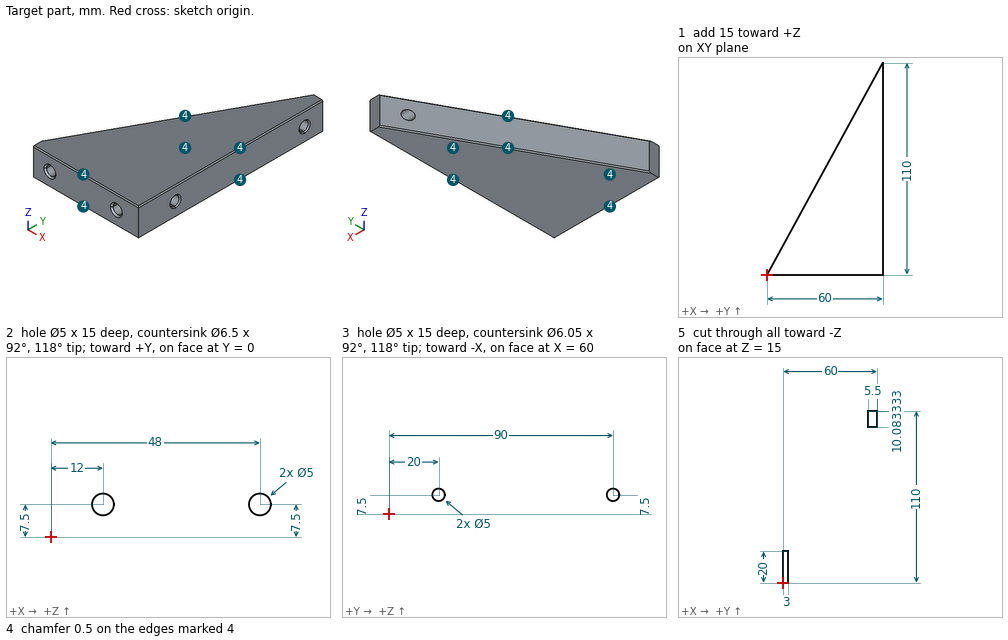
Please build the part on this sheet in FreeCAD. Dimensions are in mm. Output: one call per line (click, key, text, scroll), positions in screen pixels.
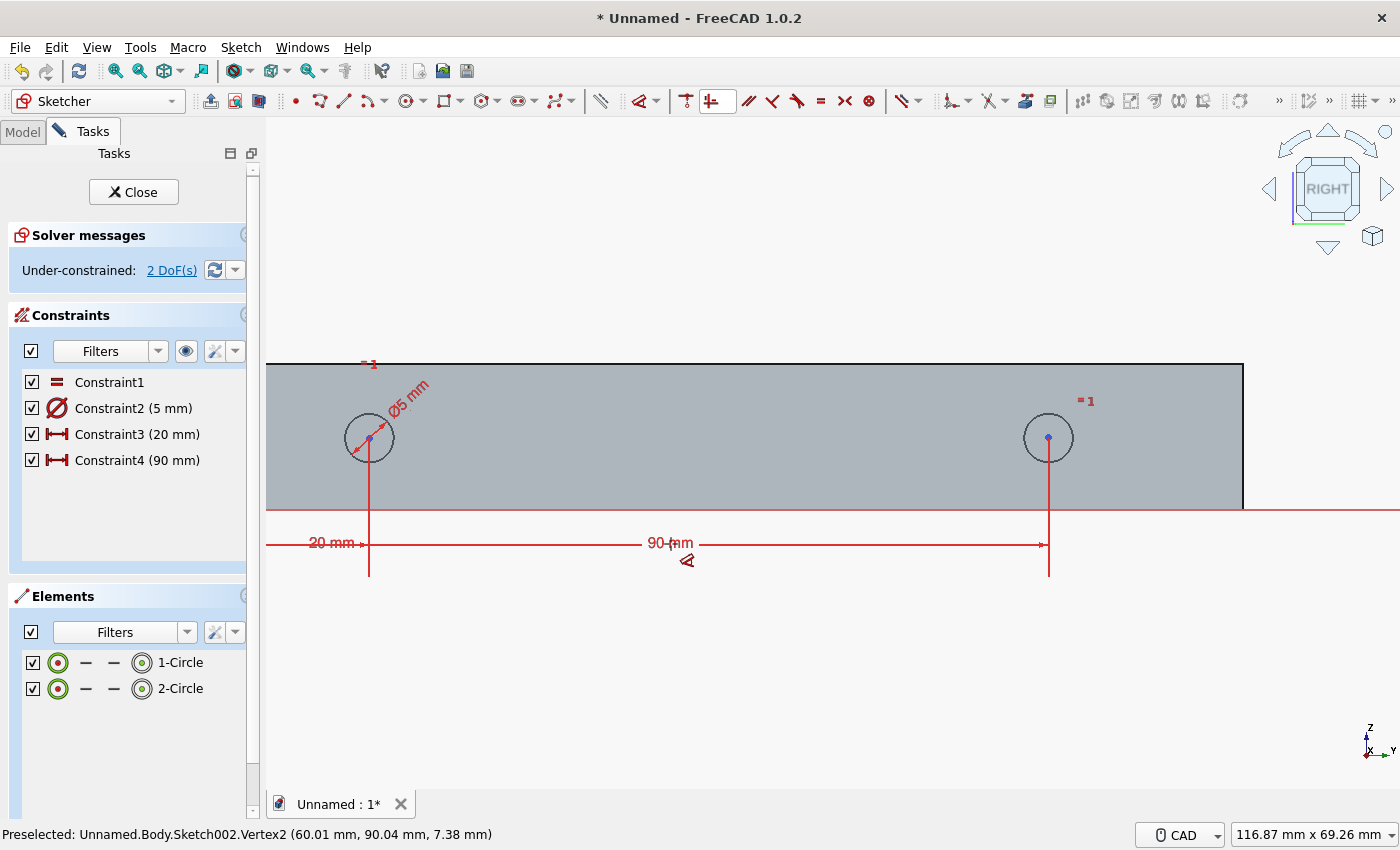
click(369, 438)
click(403, 474)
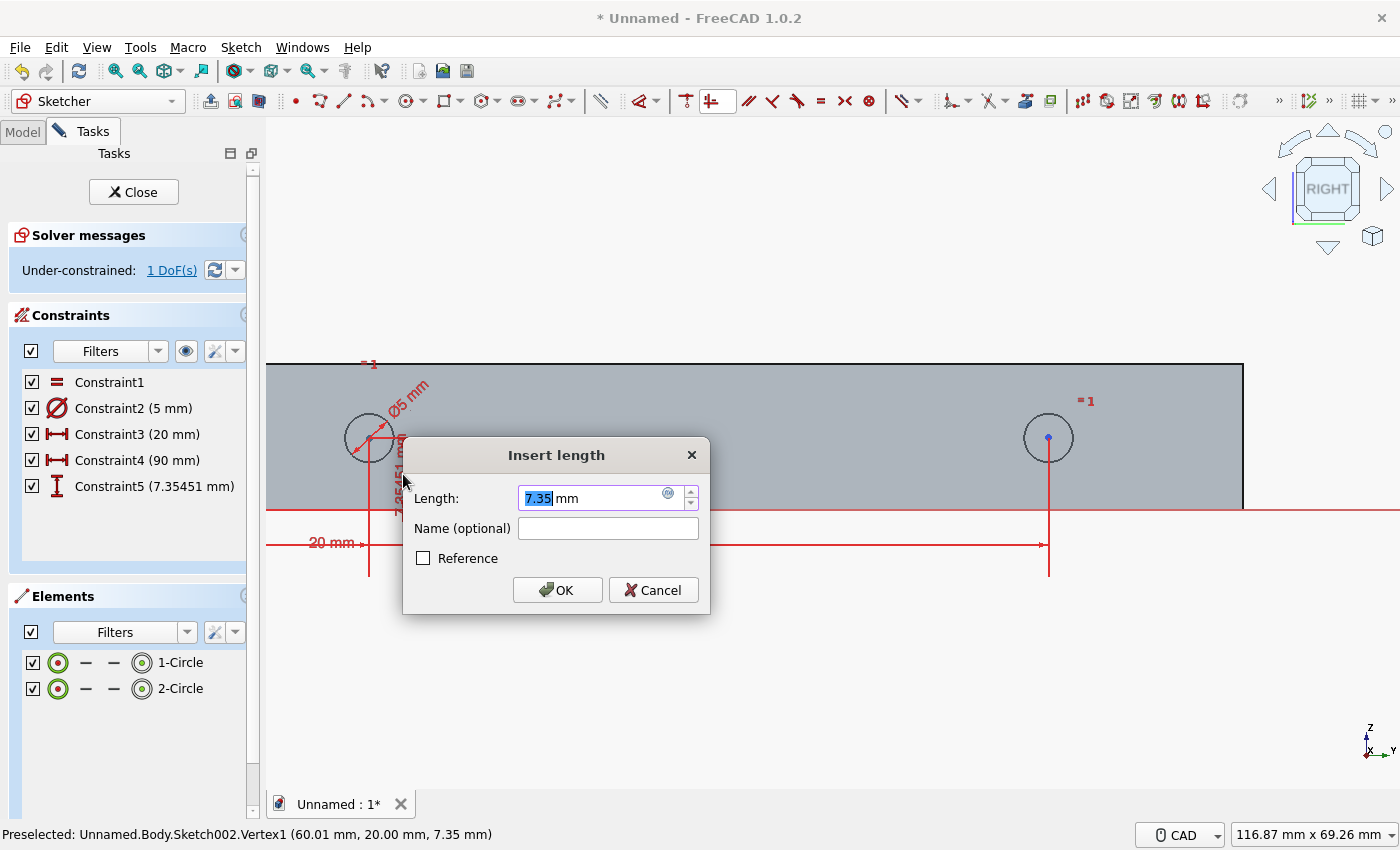
text(7.5)
key(Return)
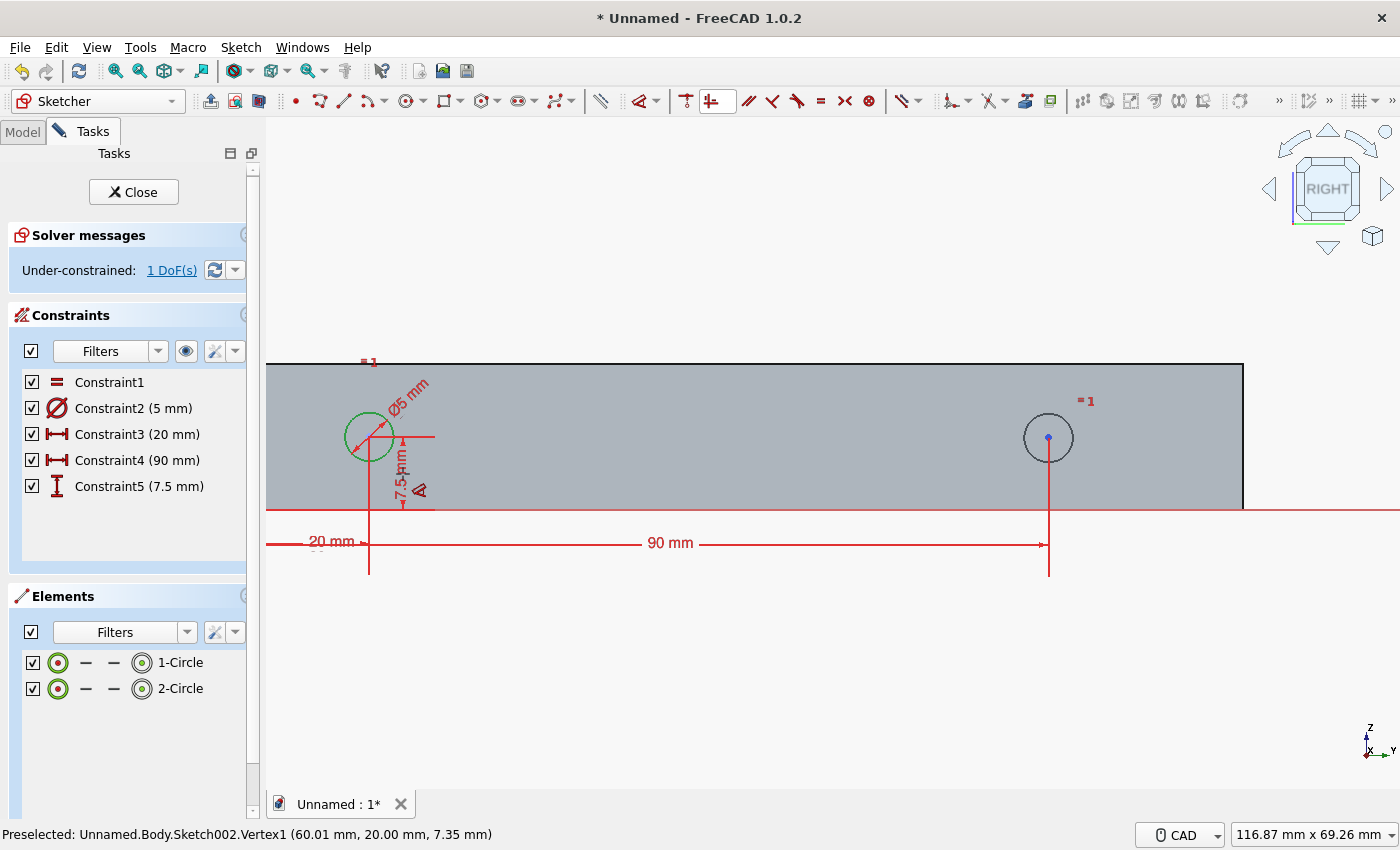
click(1049, 438)
click(1083, 474)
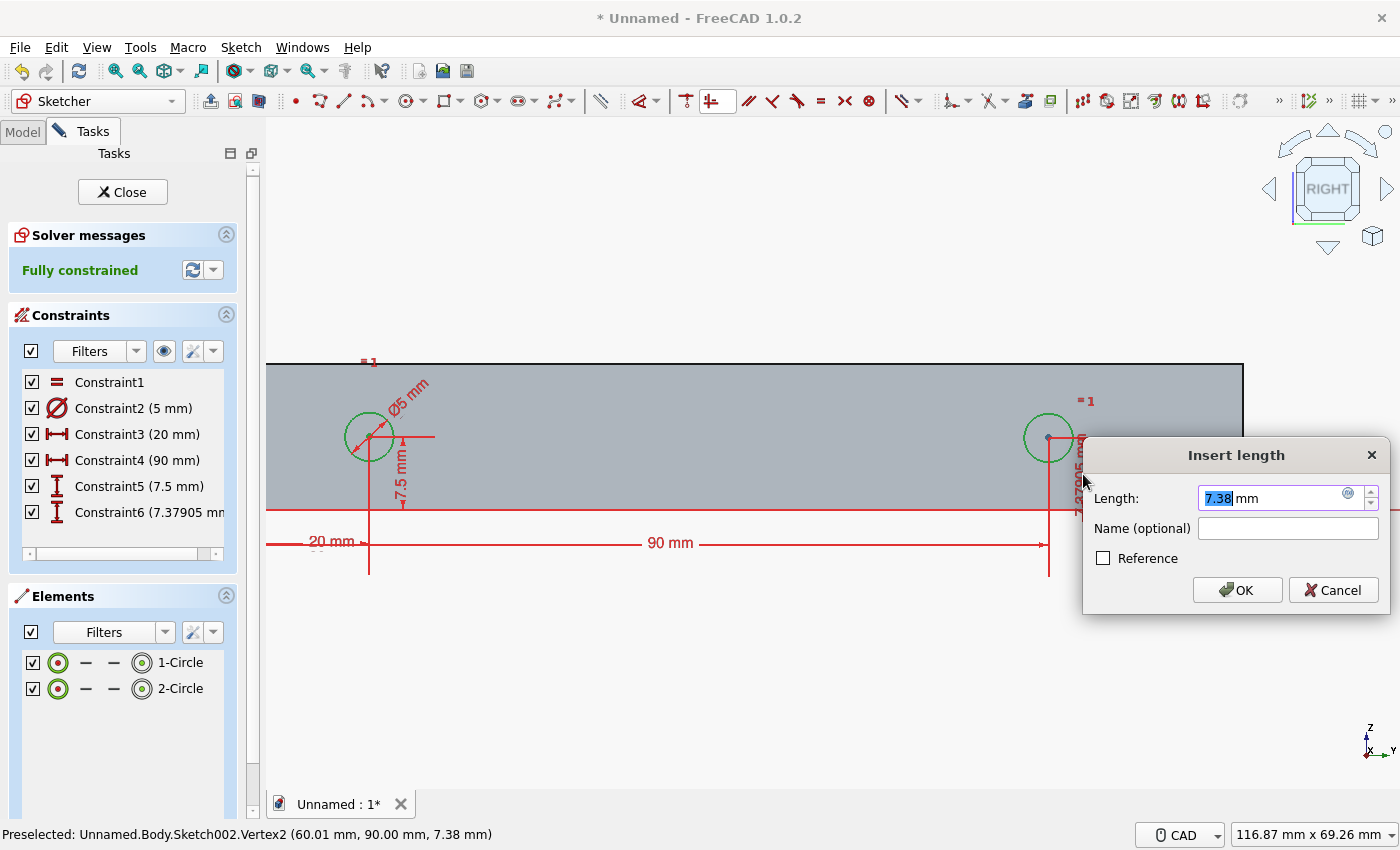
text(7.5)
key(Return)
key(Escape)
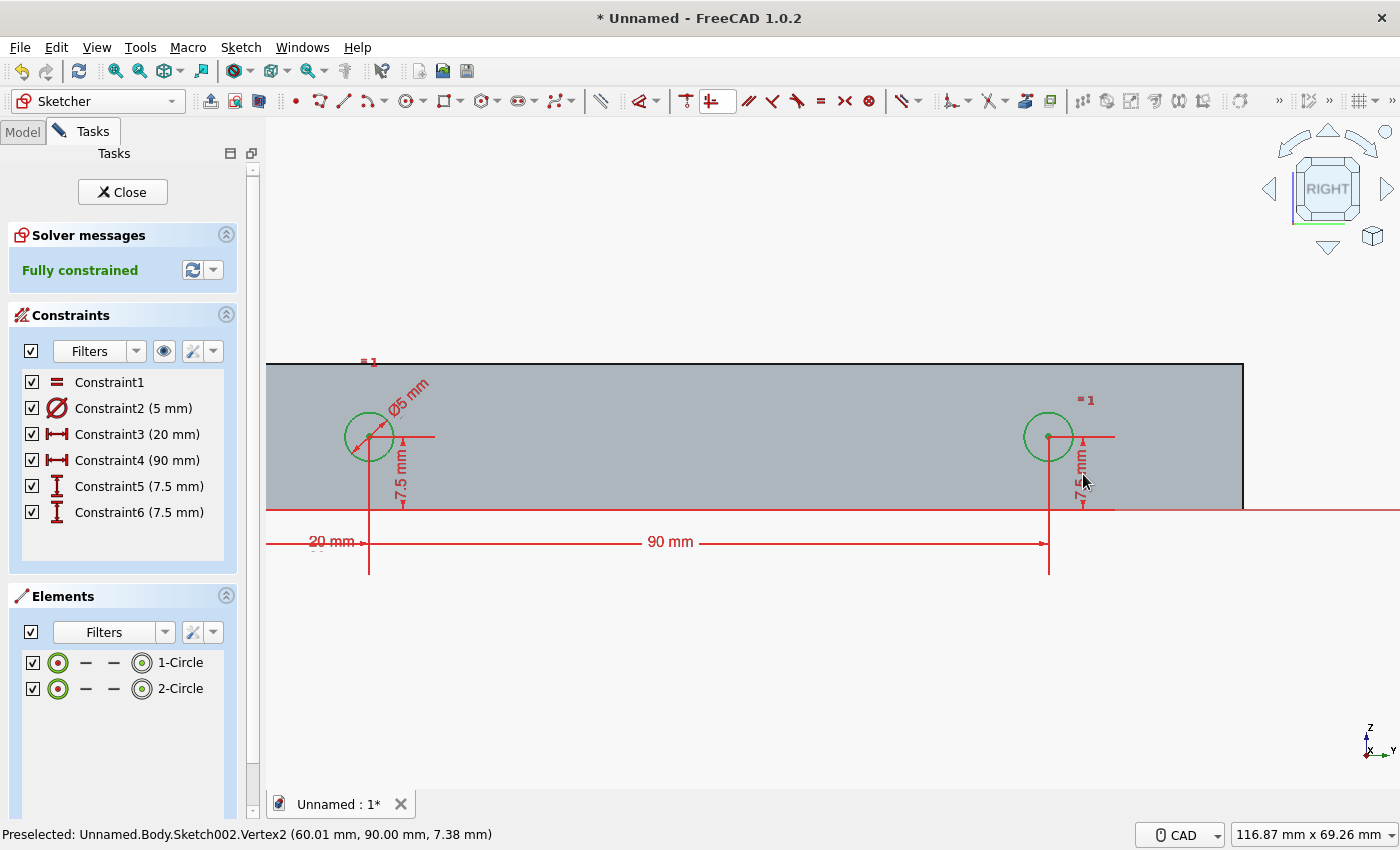
click(123, 192)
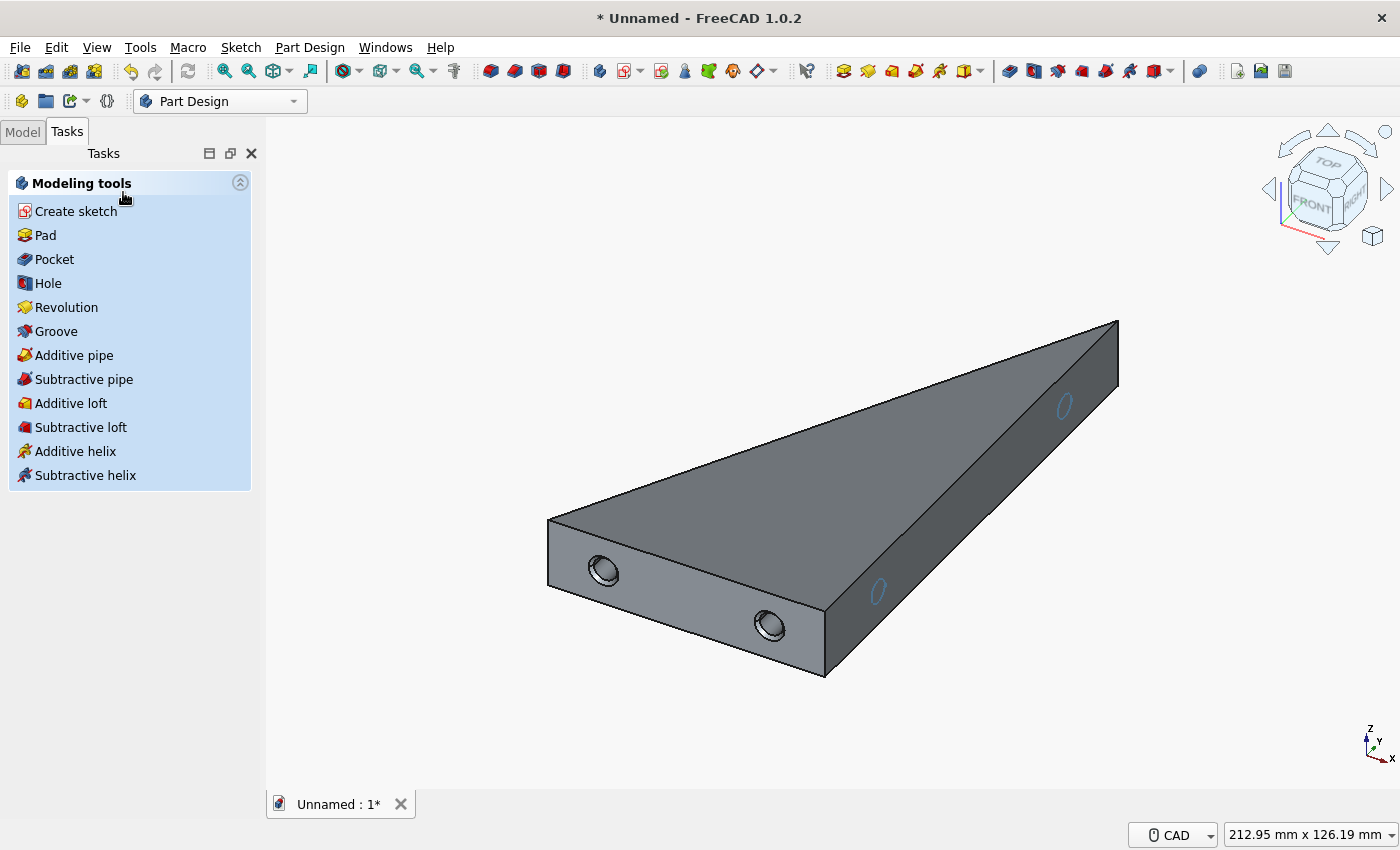
click(1034, 72)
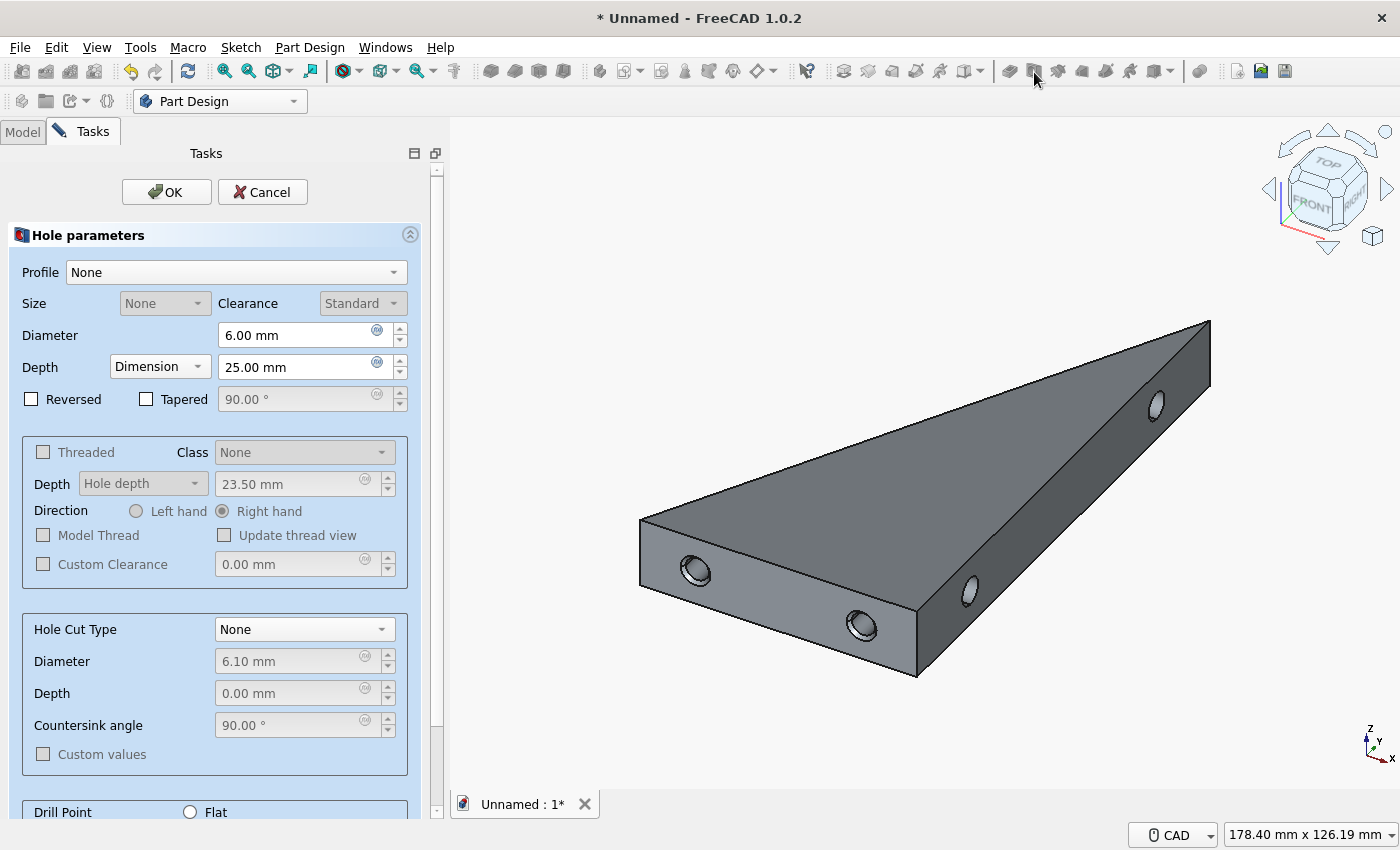
triple_click(305, 335)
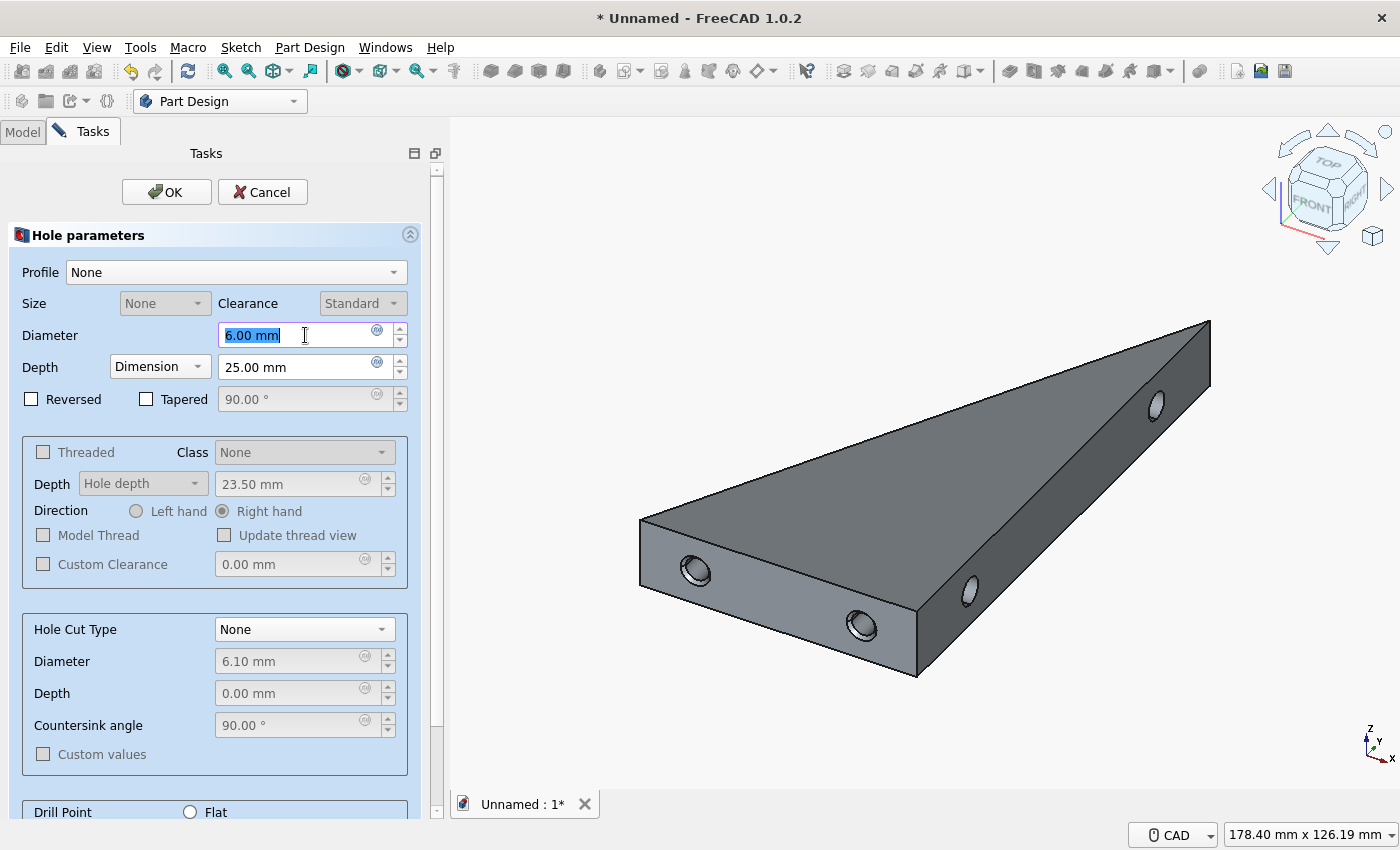
text(5)
key(Tab)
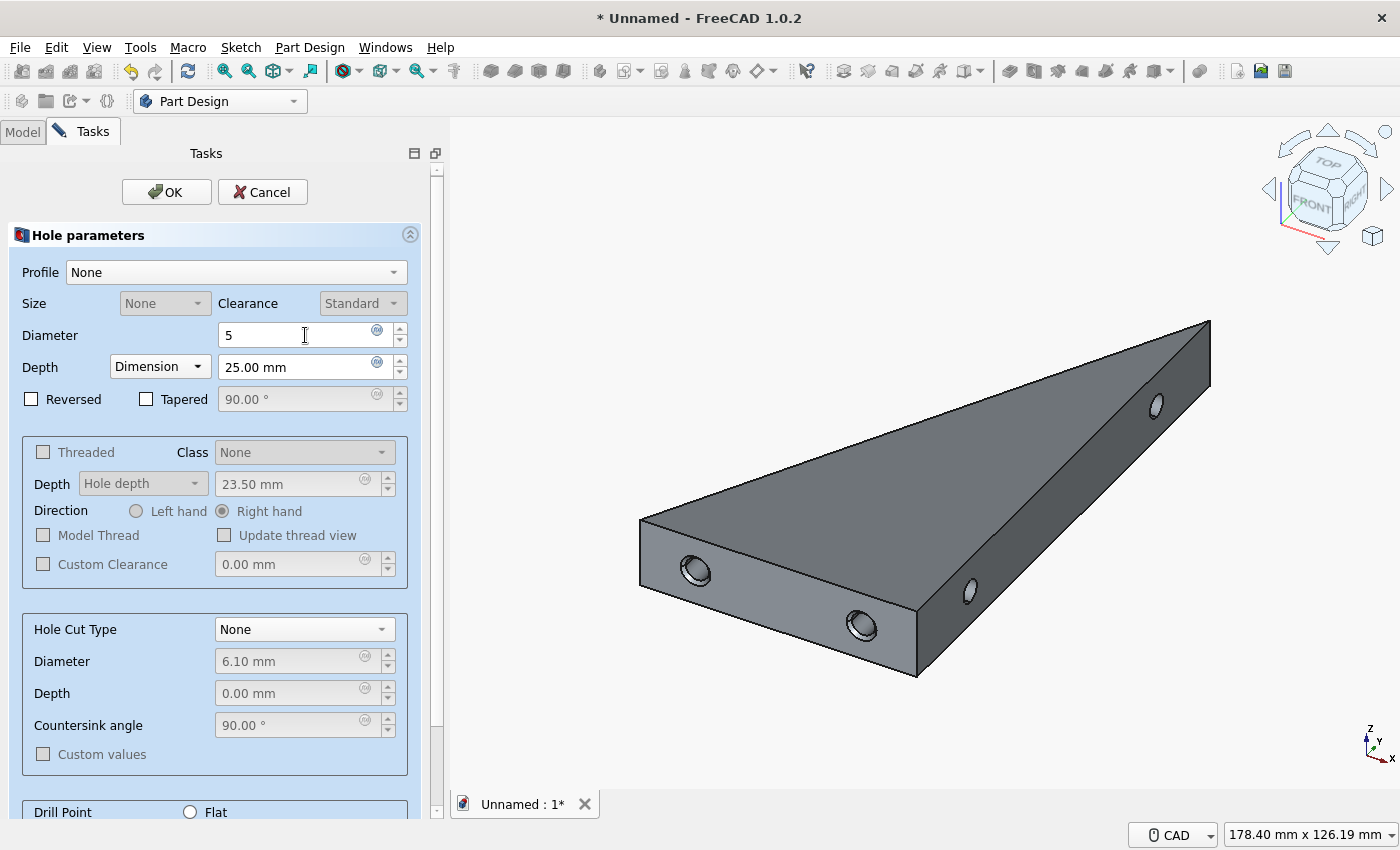
triple_click(305, 367)